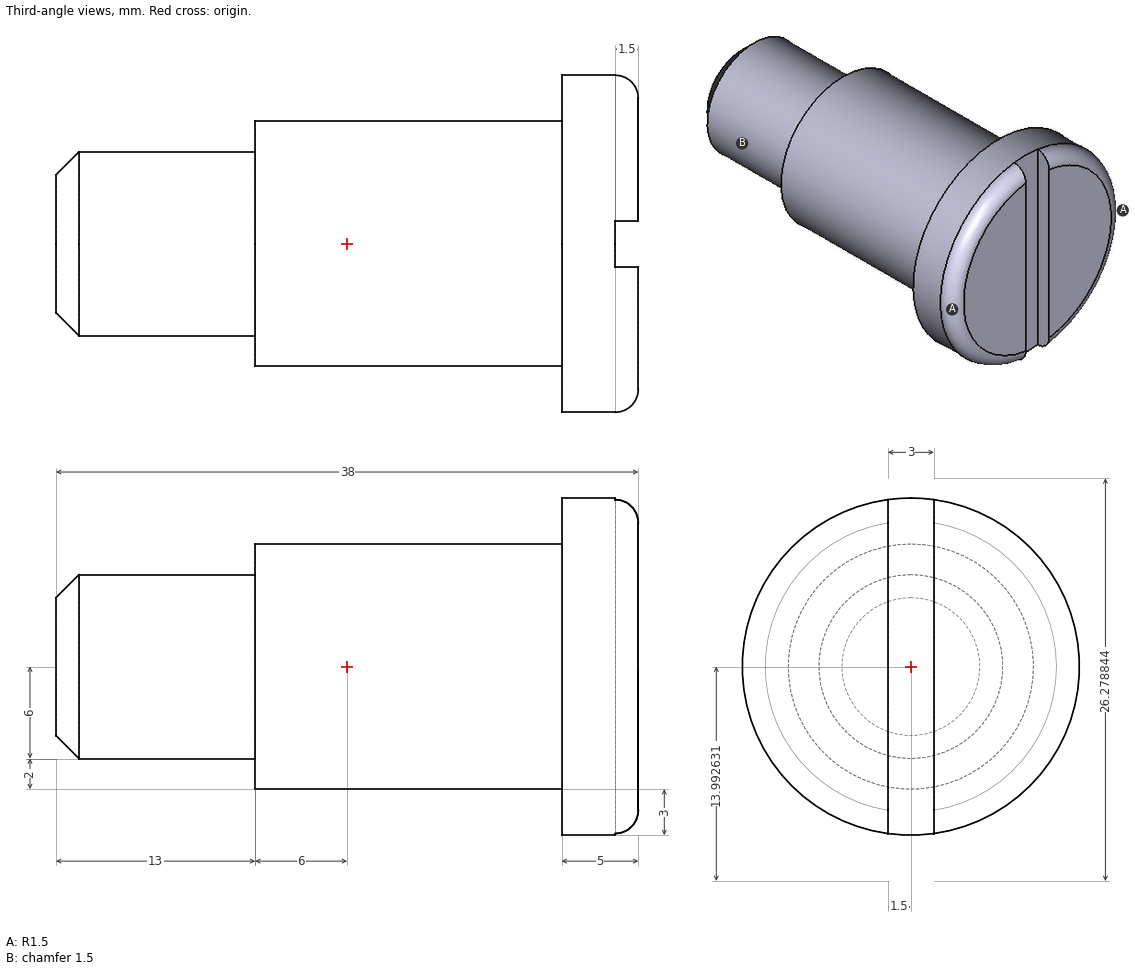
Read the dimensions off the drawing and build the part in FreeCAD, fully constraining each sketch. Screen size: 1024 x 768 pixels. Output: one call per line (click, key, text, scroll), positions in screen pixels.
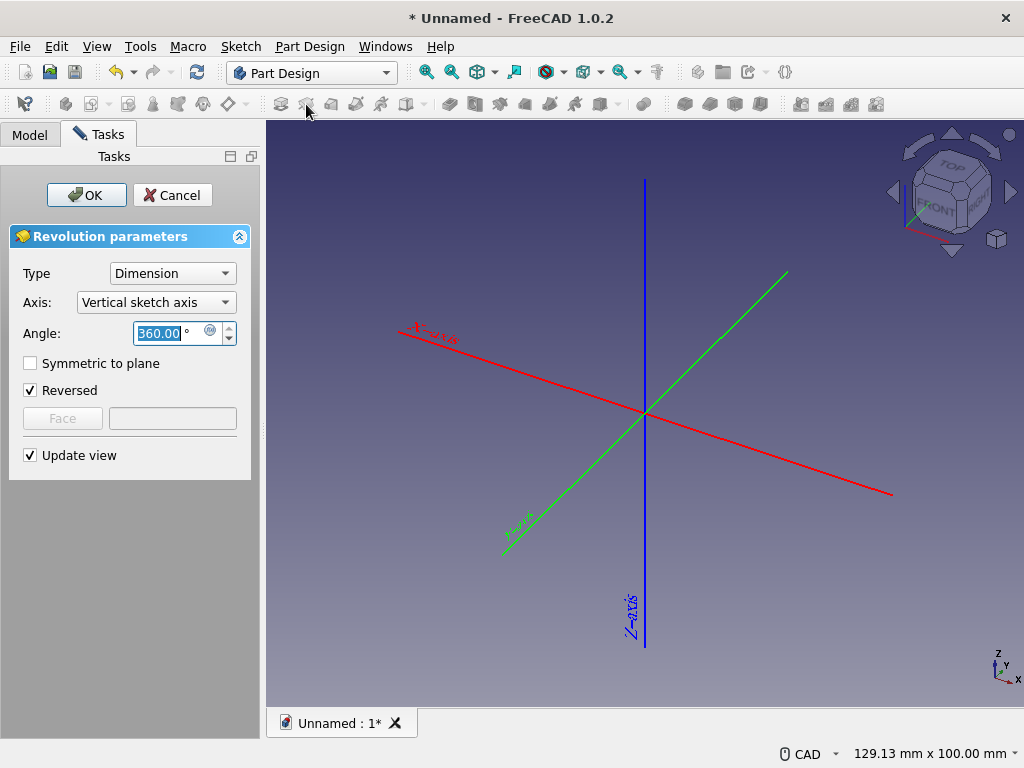
click(157, 302)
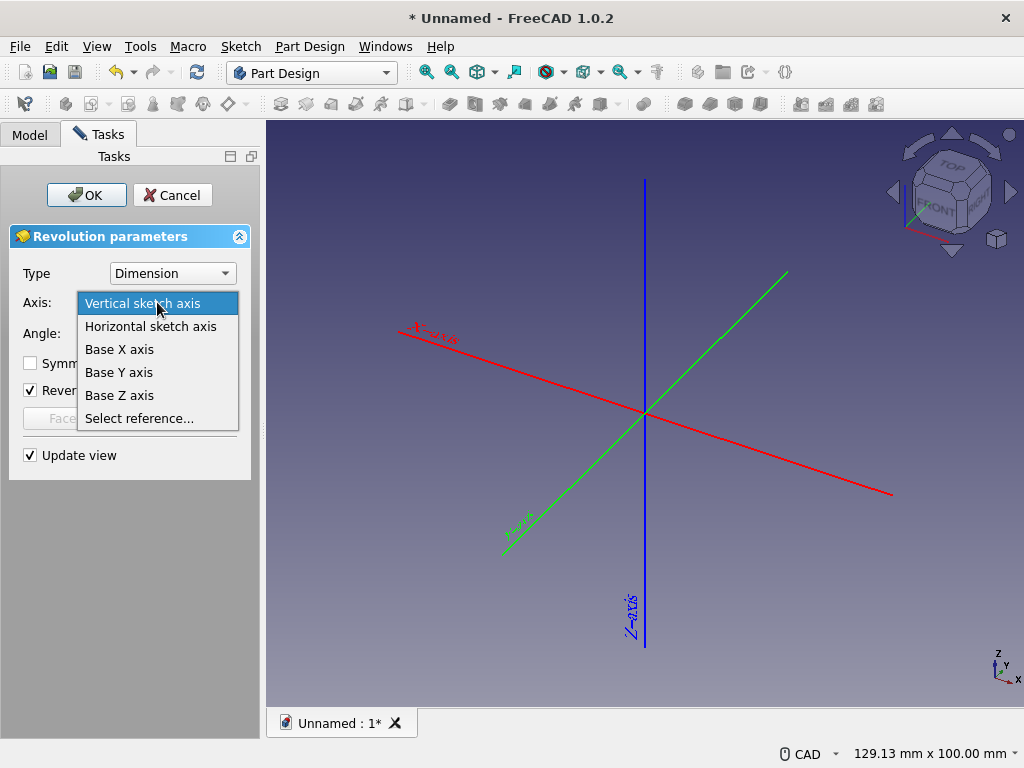
click(156, 326)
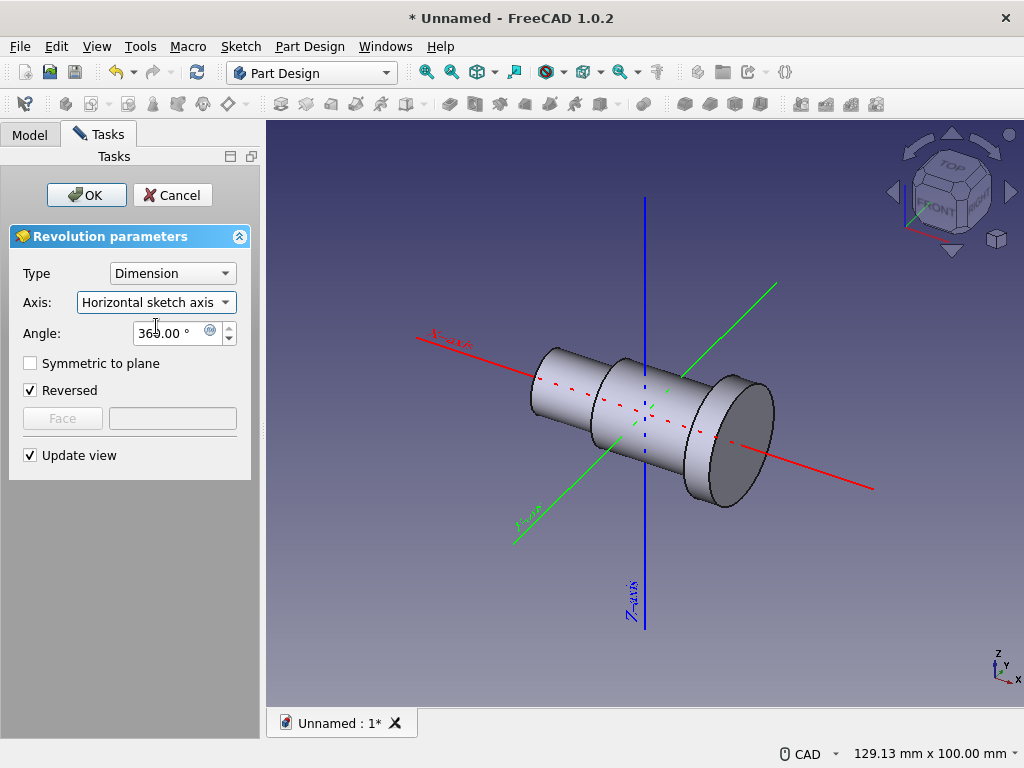
click(87, 195)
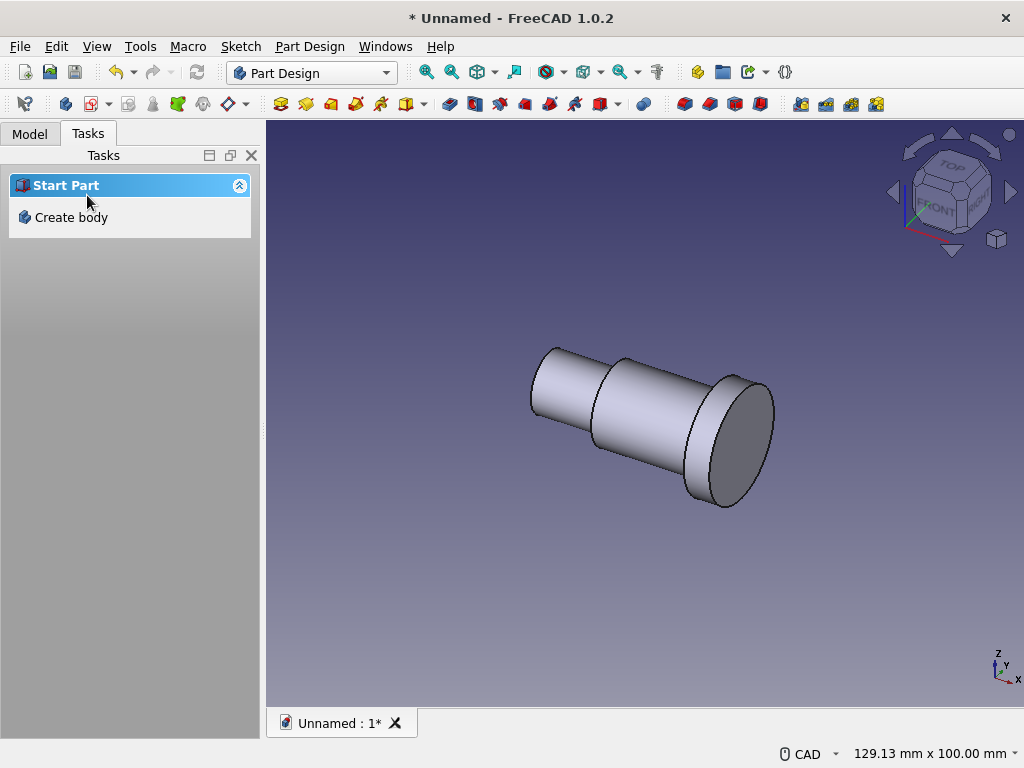
key(v)
key(f)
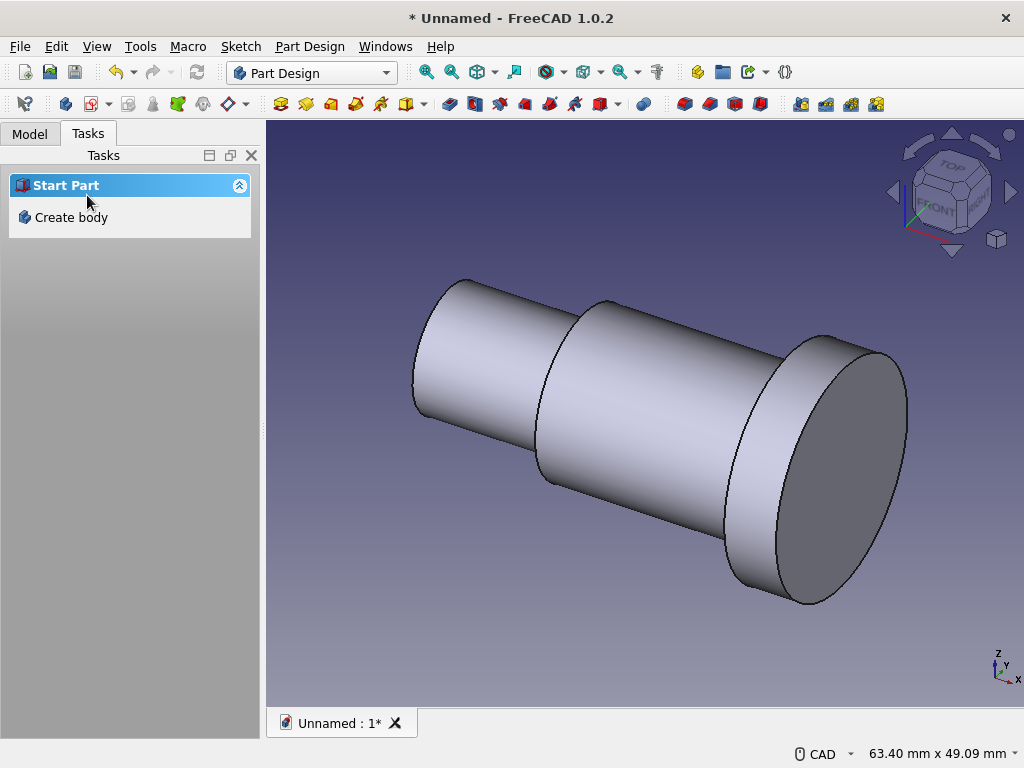
click(842, 478)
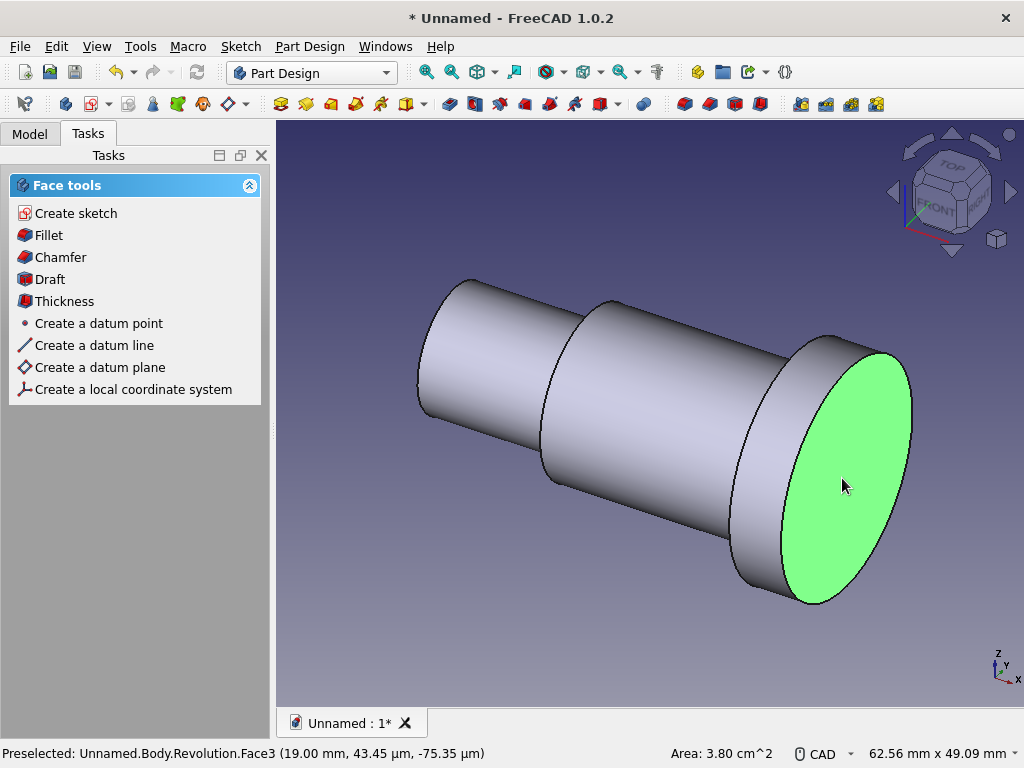
click(90, 104)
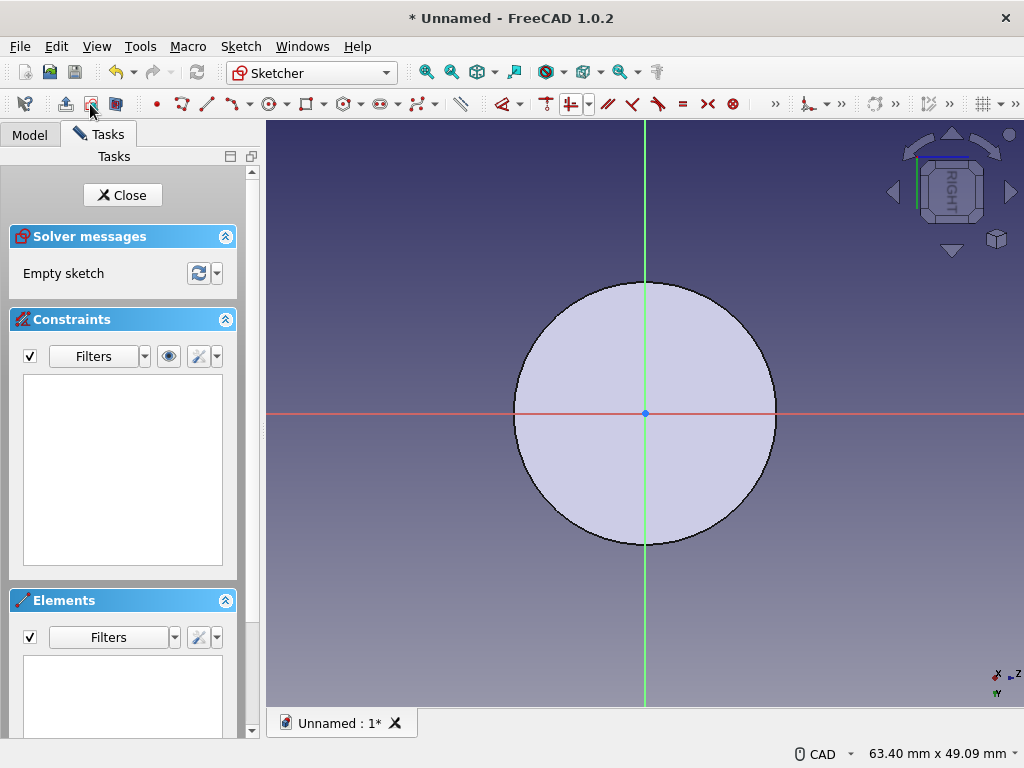
click(306, 104)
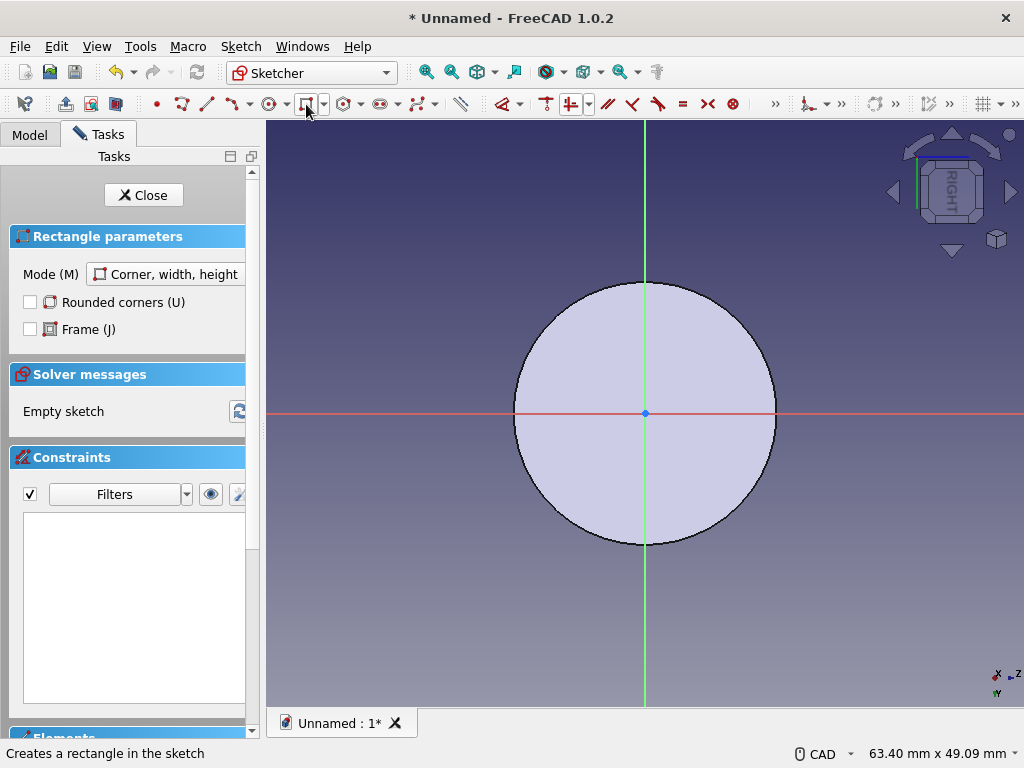
click(478, 396)
move(792, 431)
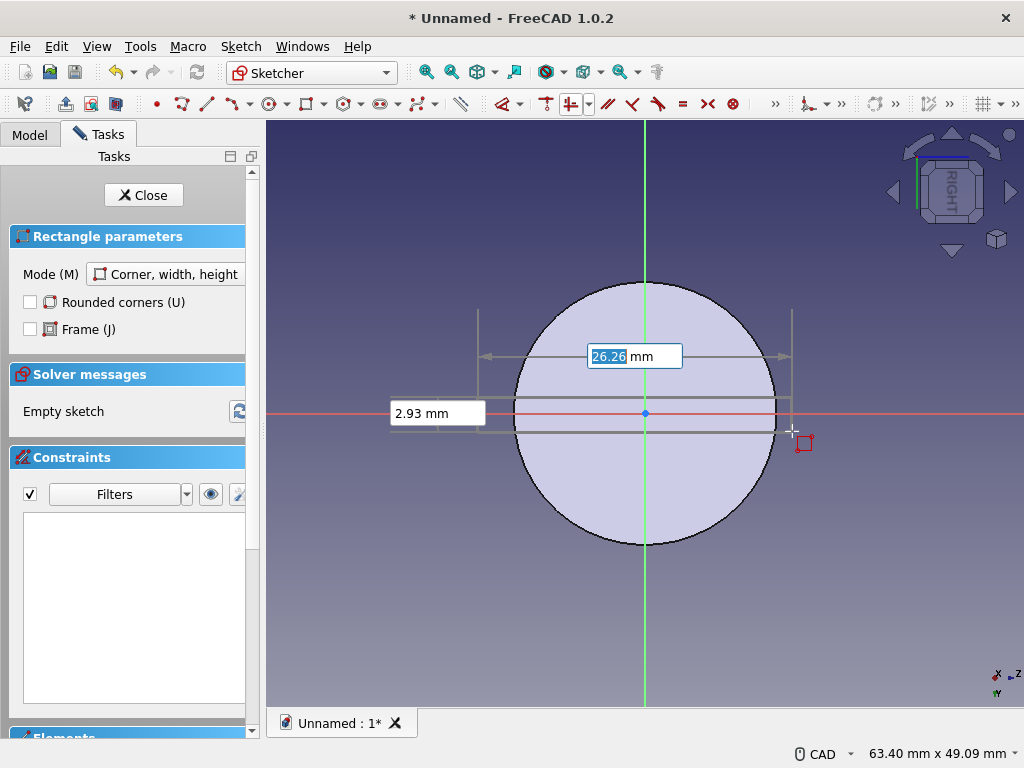
text(26.278844)
key(Tab)
text(3)
key(Return)
key(Escape)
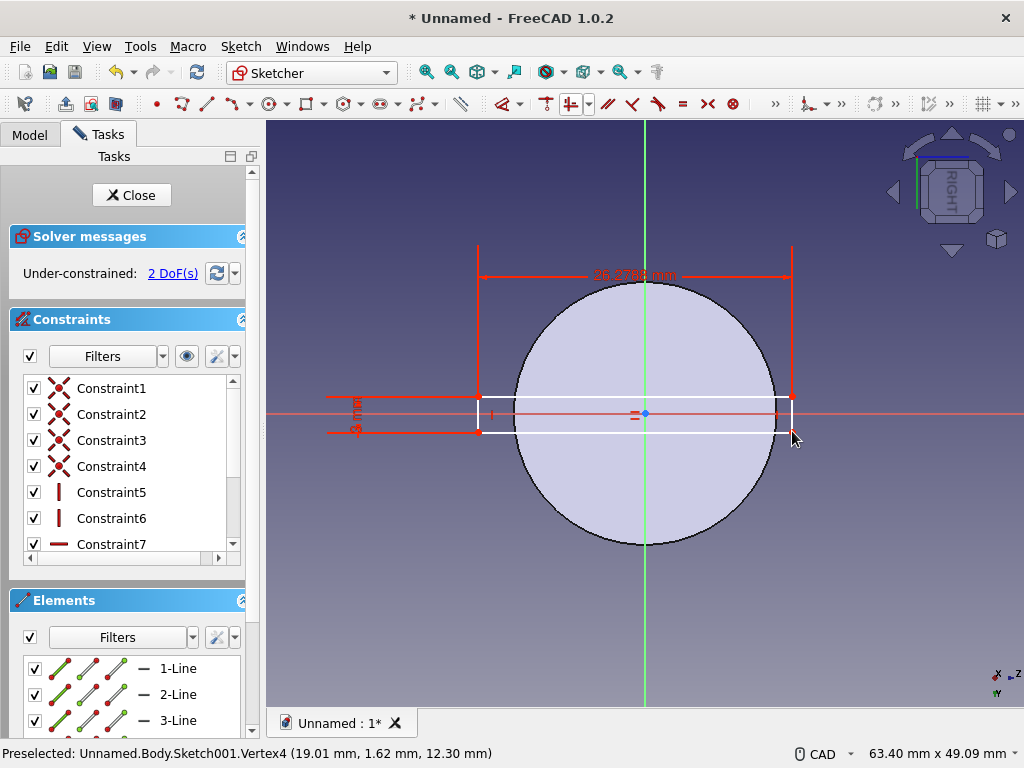
click(502, 104)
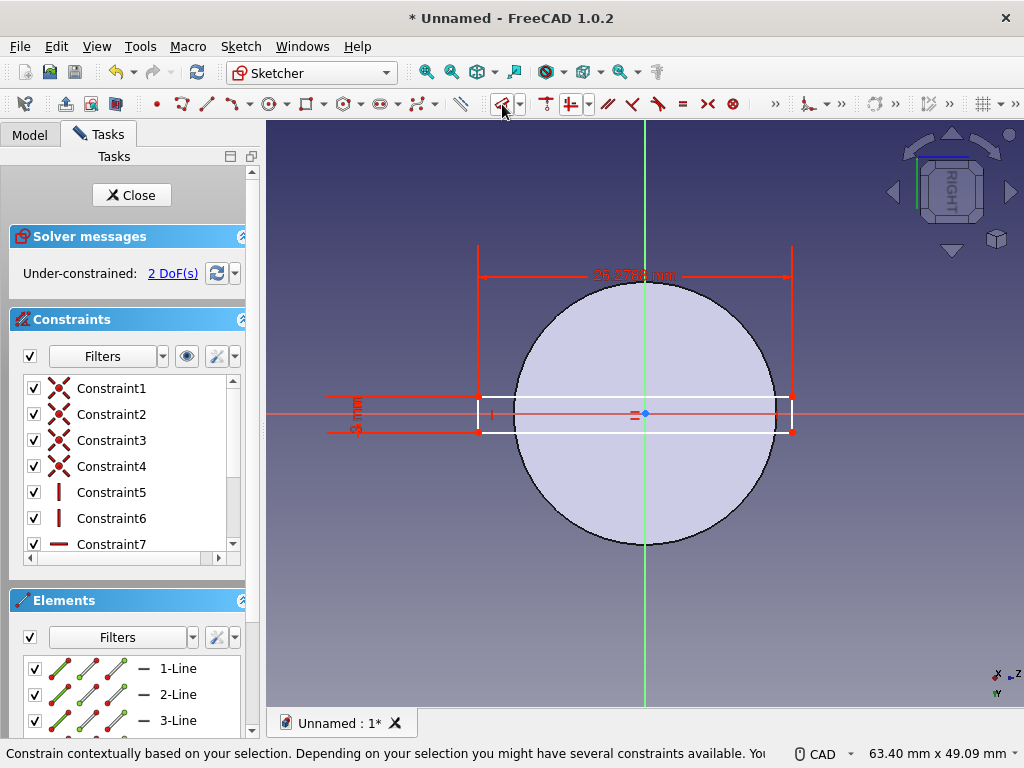
scroll(478, 397, up, 4)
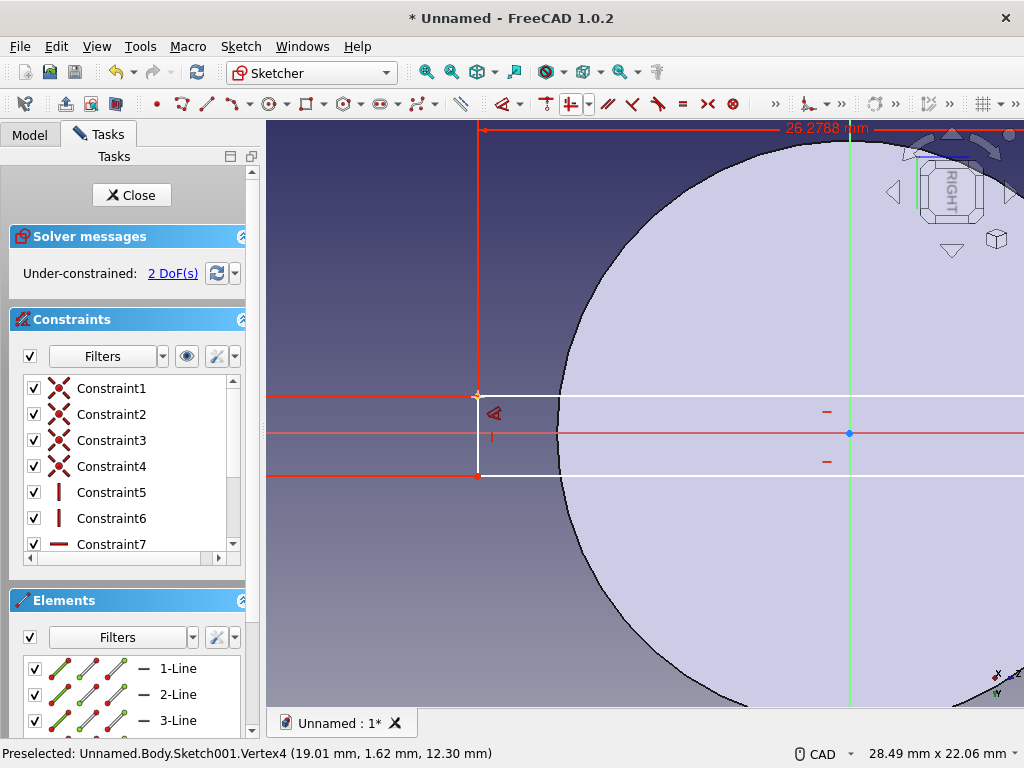
click(478, 396)
click(444, 415)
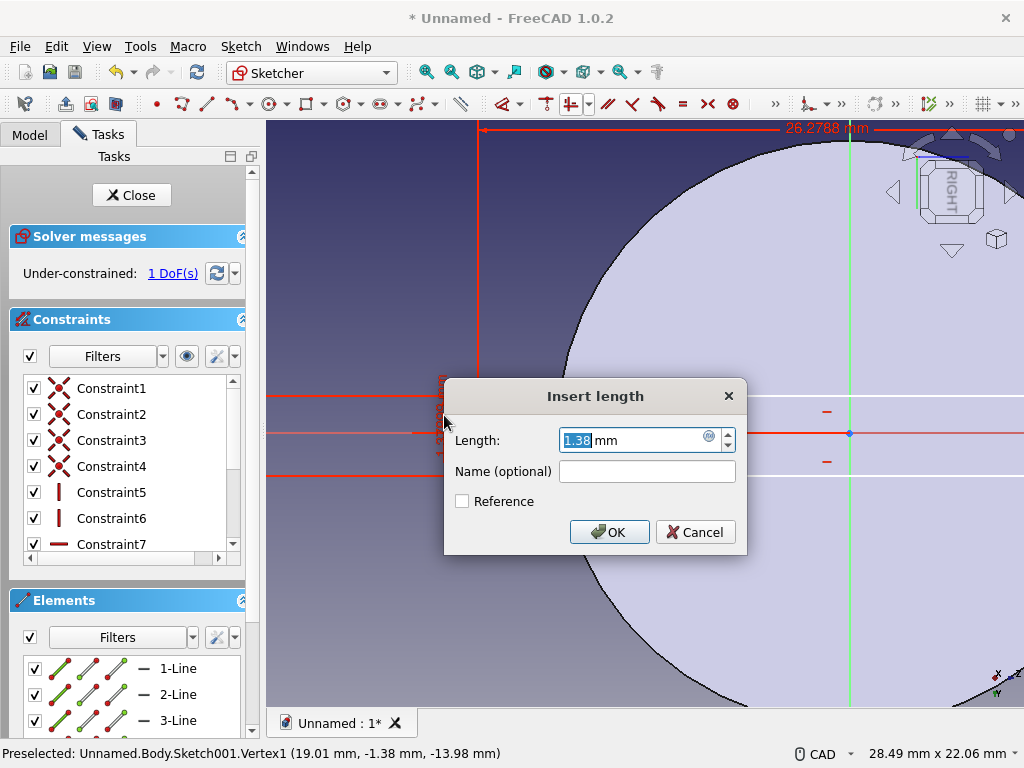
text(1.5)
key(Return)